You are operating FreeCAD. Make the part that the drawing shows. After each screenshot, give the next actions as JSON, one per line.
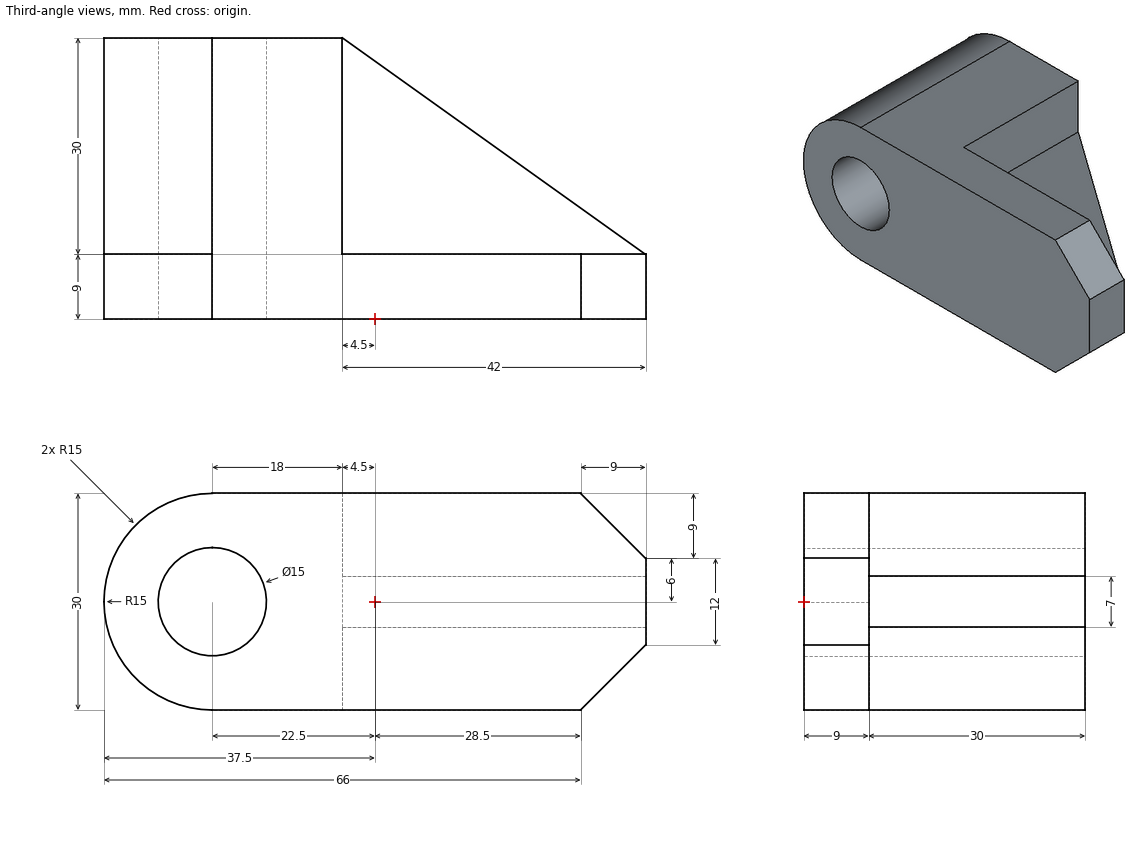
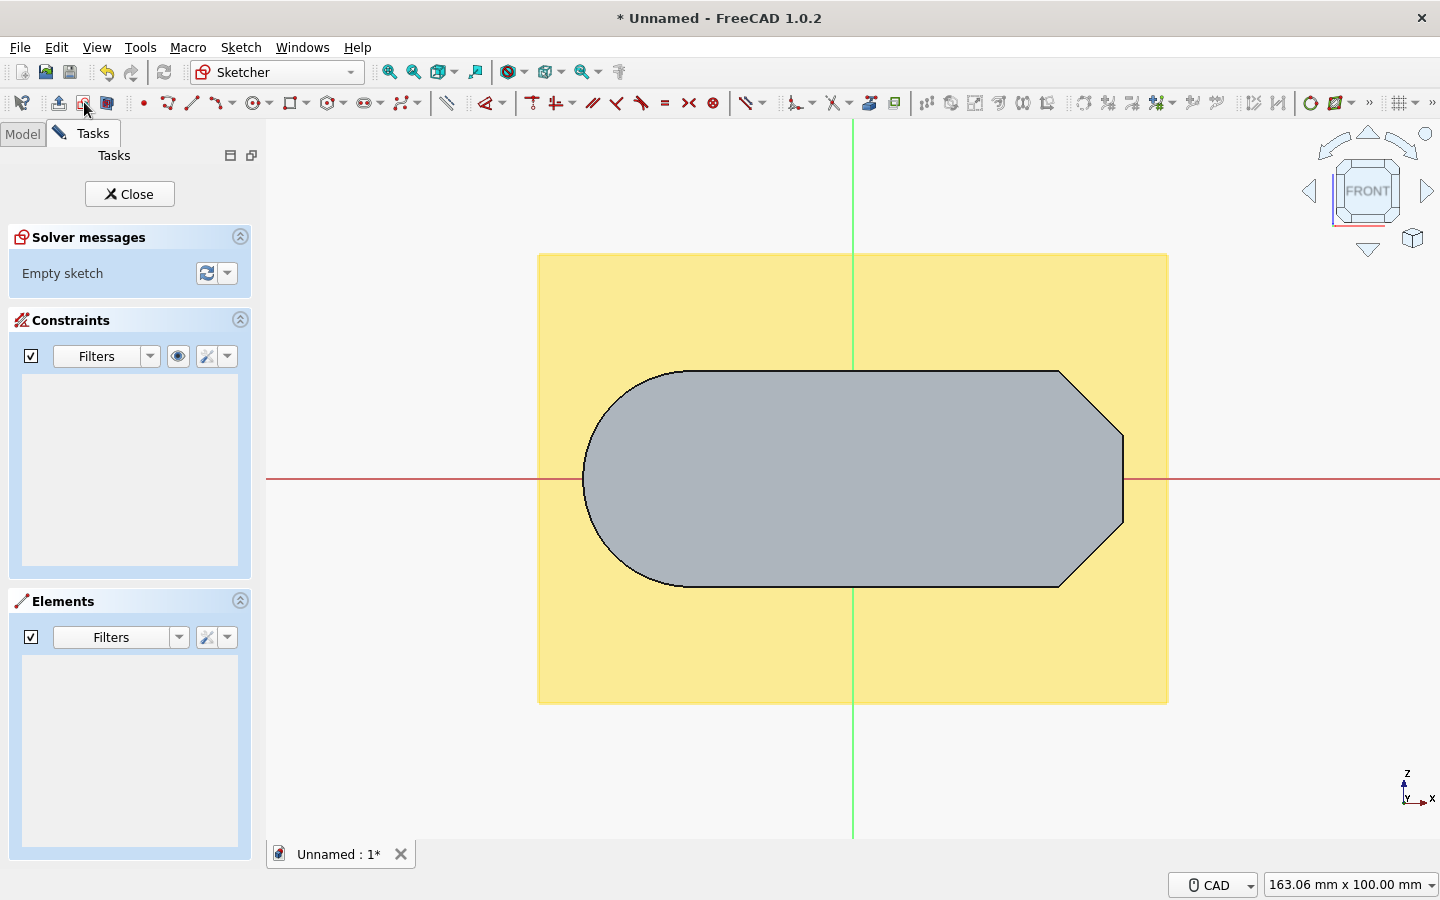
{"action": "left_click", "coordinate": [108, 104]}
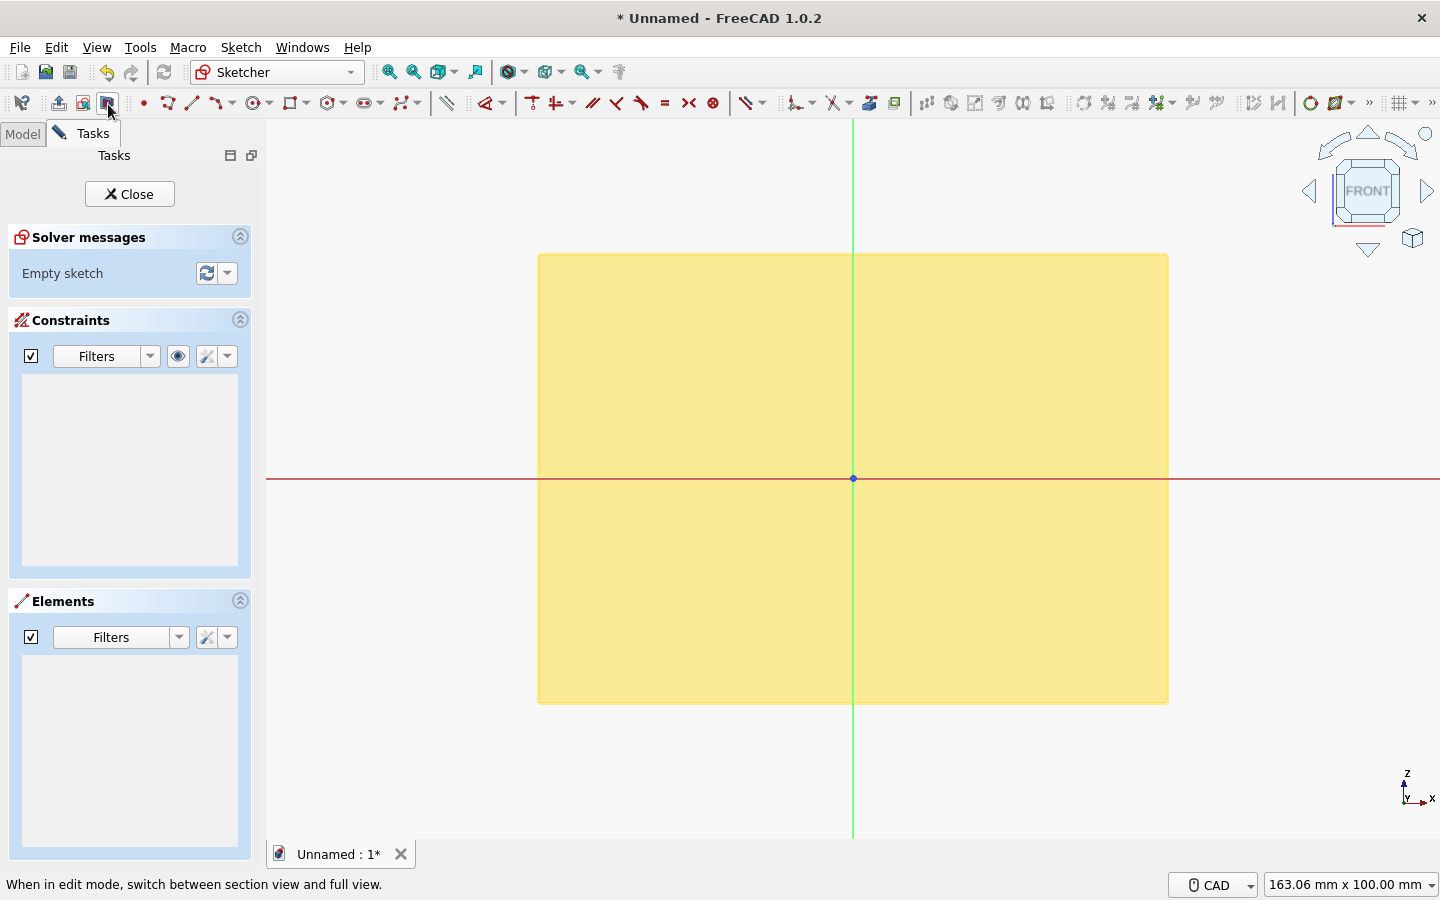
{"action": "scroll", "coordinate": [664, 479], "scroll_direction": "up", "scroll_amount": 4}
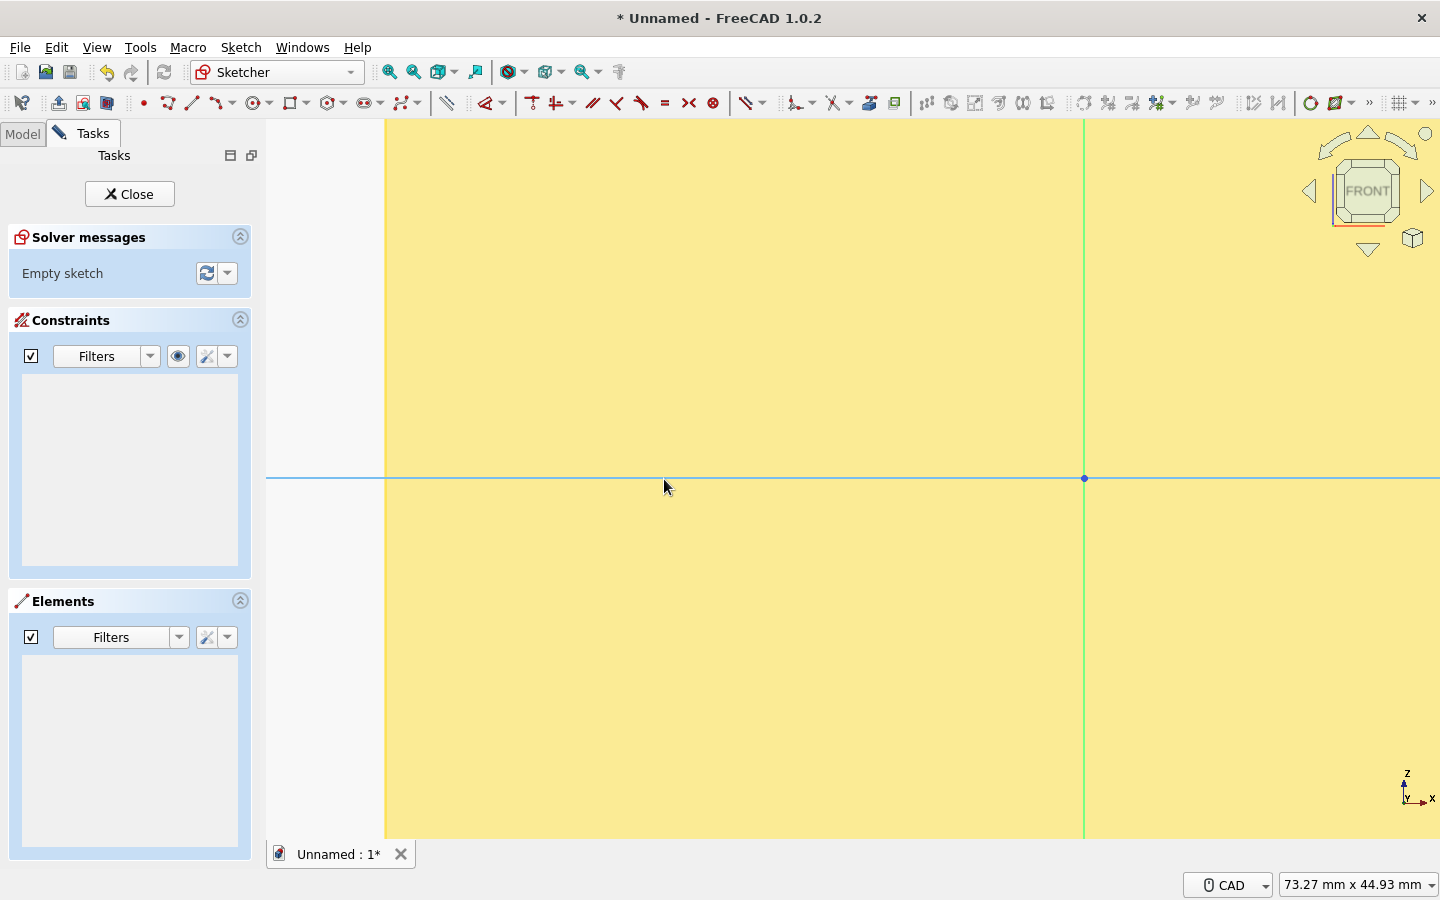
{"action": "left_click", "coordinate": [168, 104]}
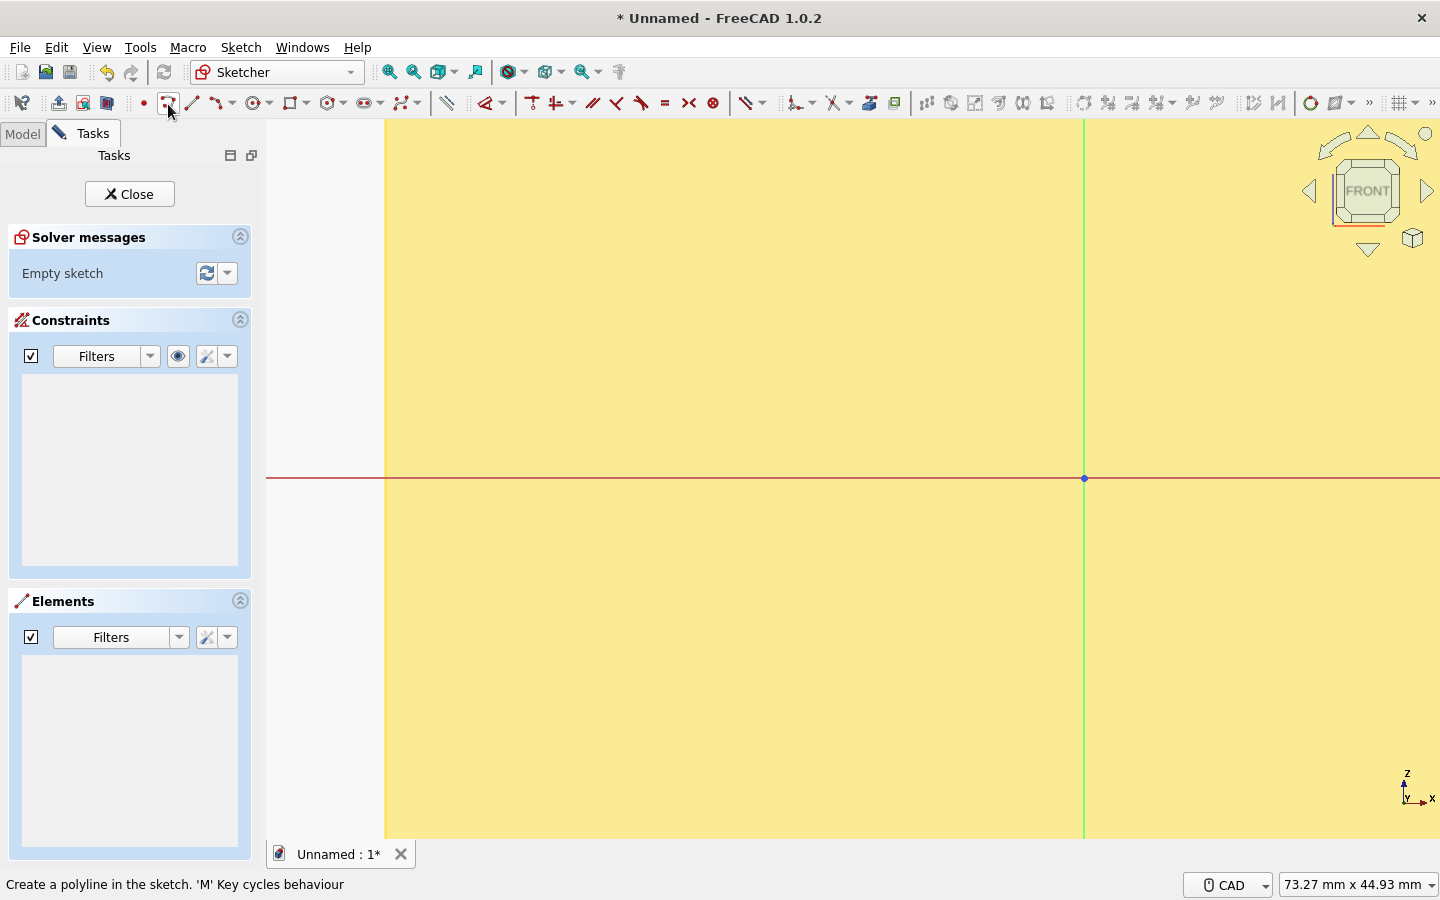
{"action": "left_click", "coordinate": [724, 238]}
{"action": "left_click", "coordinate": [1012, 238]}
{"action": "left_click", "coordinate": [1012, 719]}
{"action": "left_click", "coordinate": [724, 719]}
{"action": "right_click", "coordinate": [724, 719]}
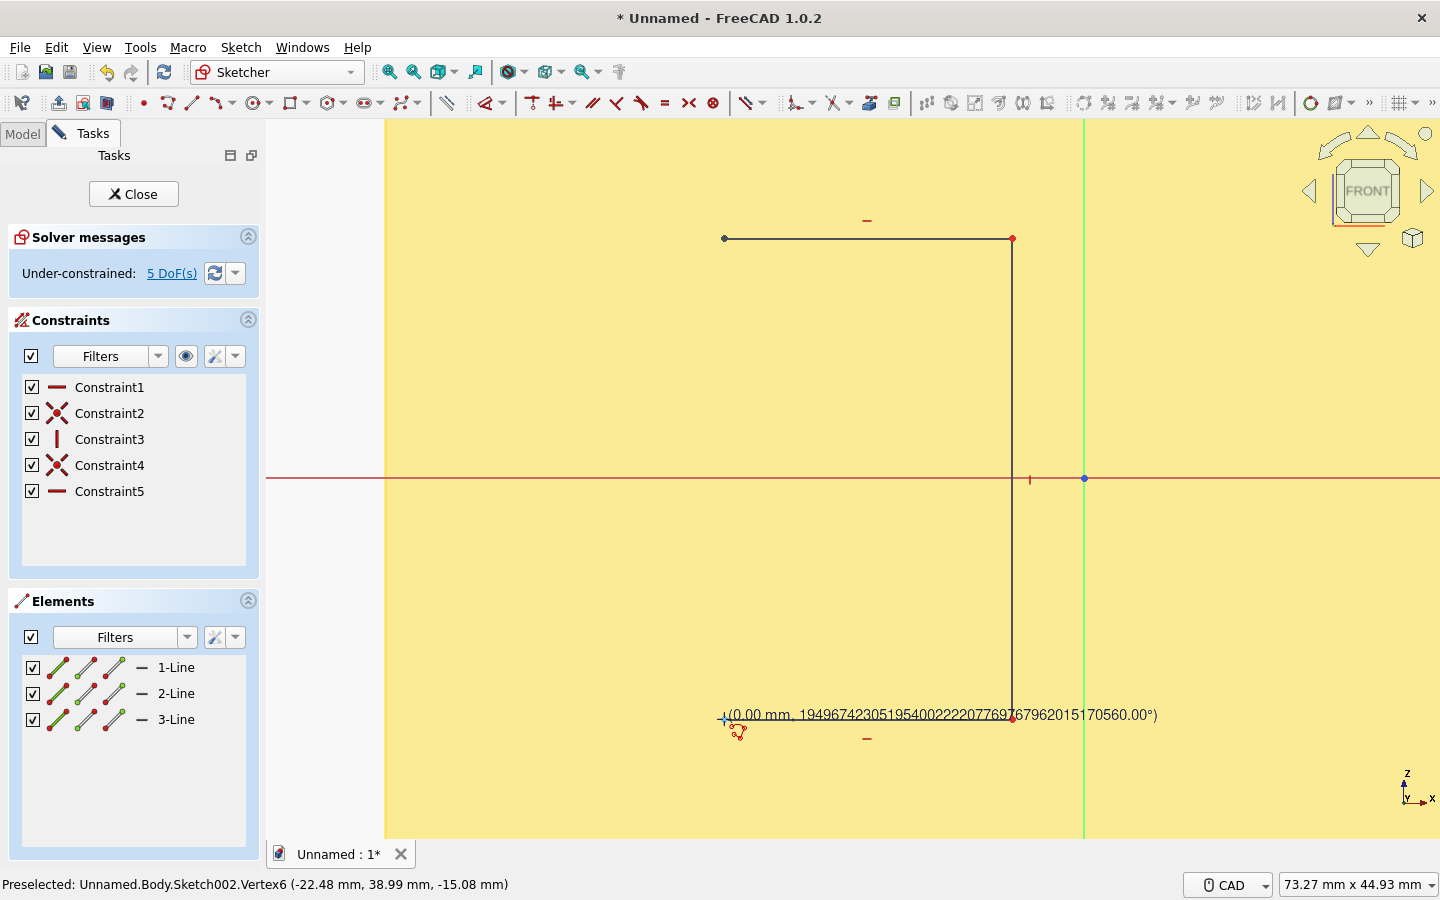
{"action": "key", "text": "g 3 a"}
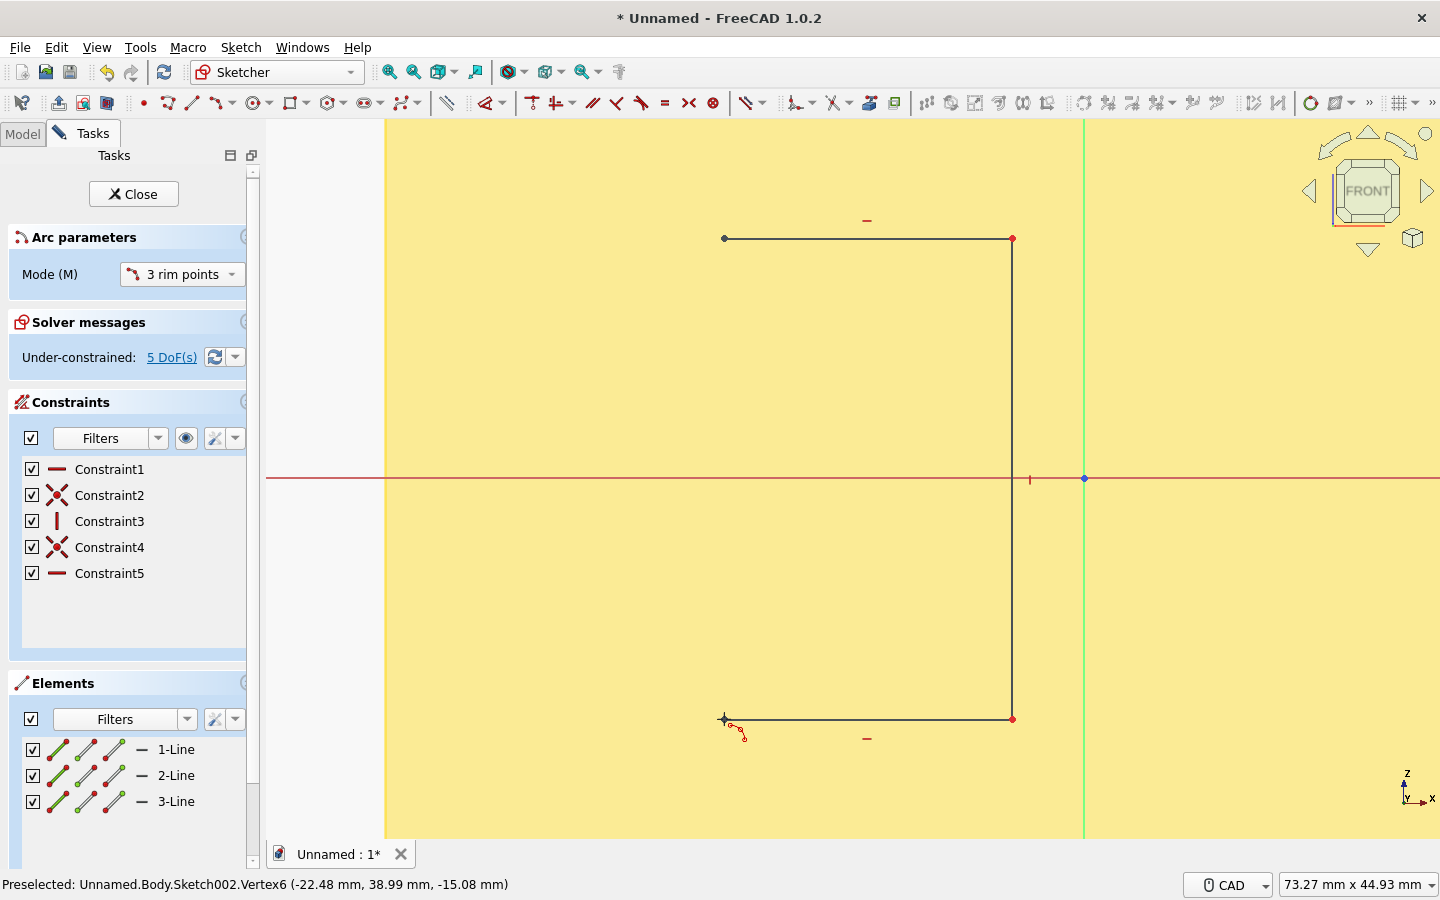
{"action": "left_click", "coordinate": [724, 720]}
{"action": "left_click", "coordinate": [724, 239]}
{"action": "left_click", "coordinate": [495, 404]}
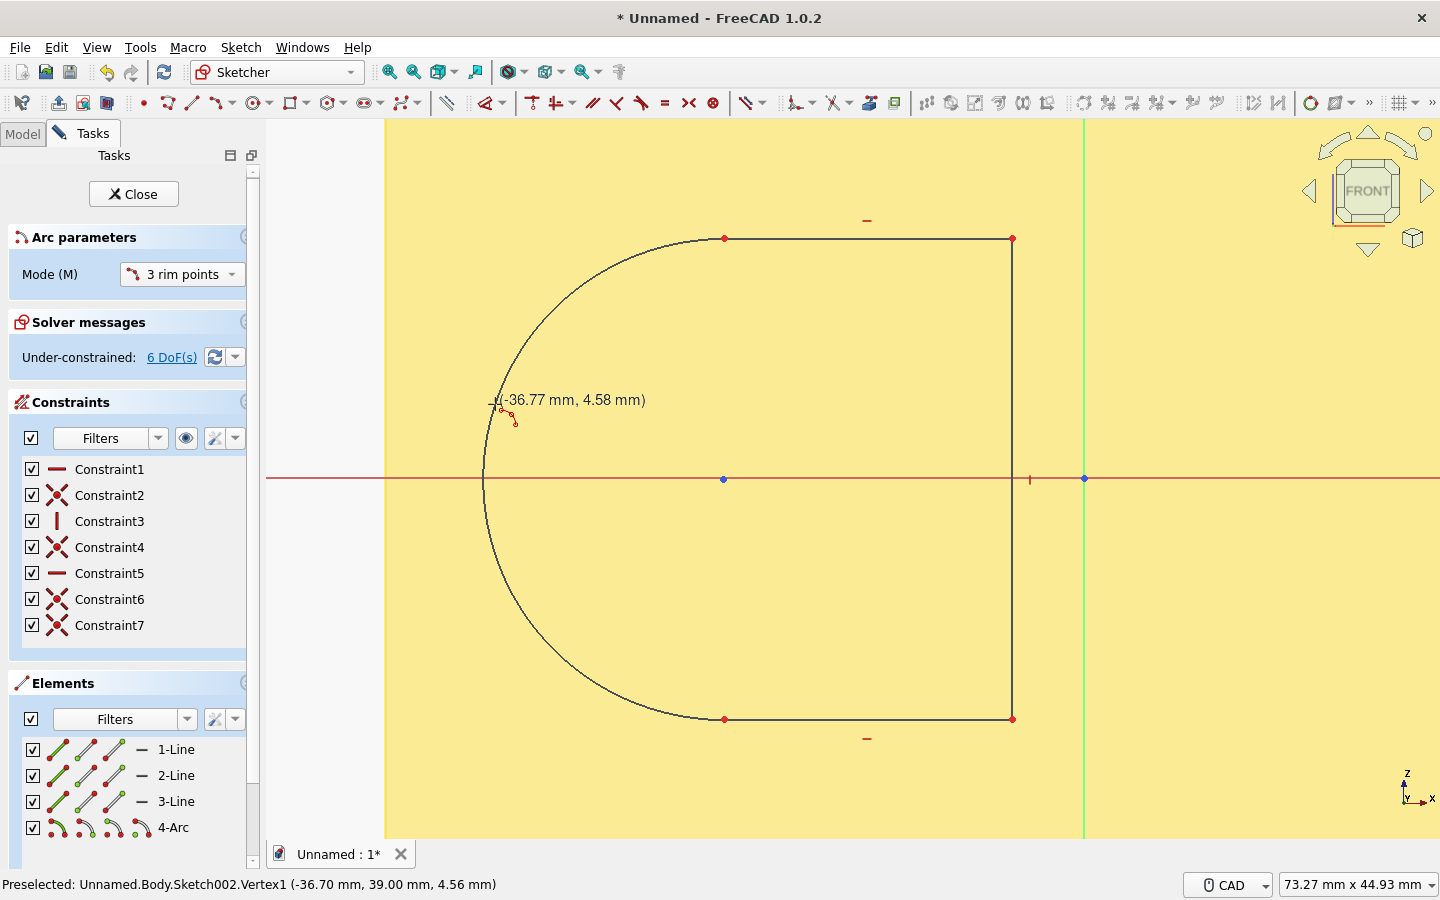
{"action": "left_click", "coordinate": [254, 104]}